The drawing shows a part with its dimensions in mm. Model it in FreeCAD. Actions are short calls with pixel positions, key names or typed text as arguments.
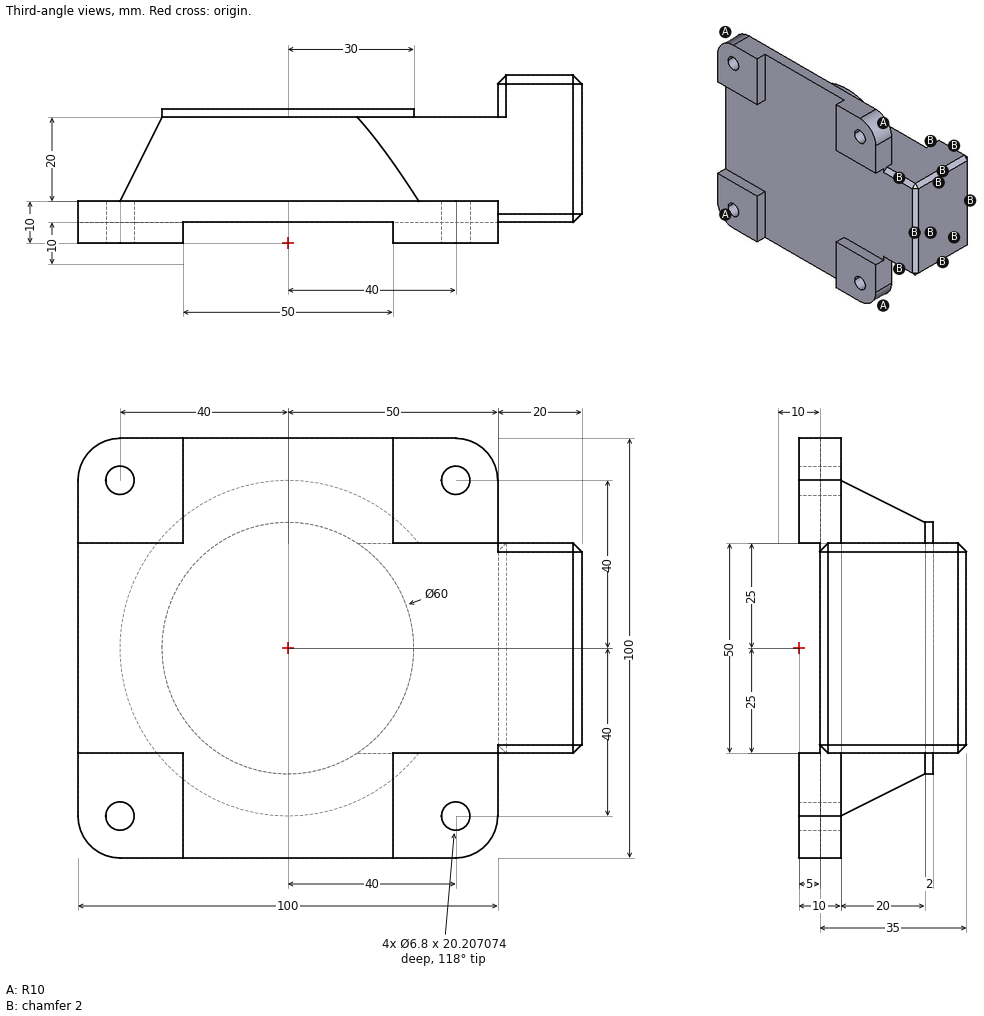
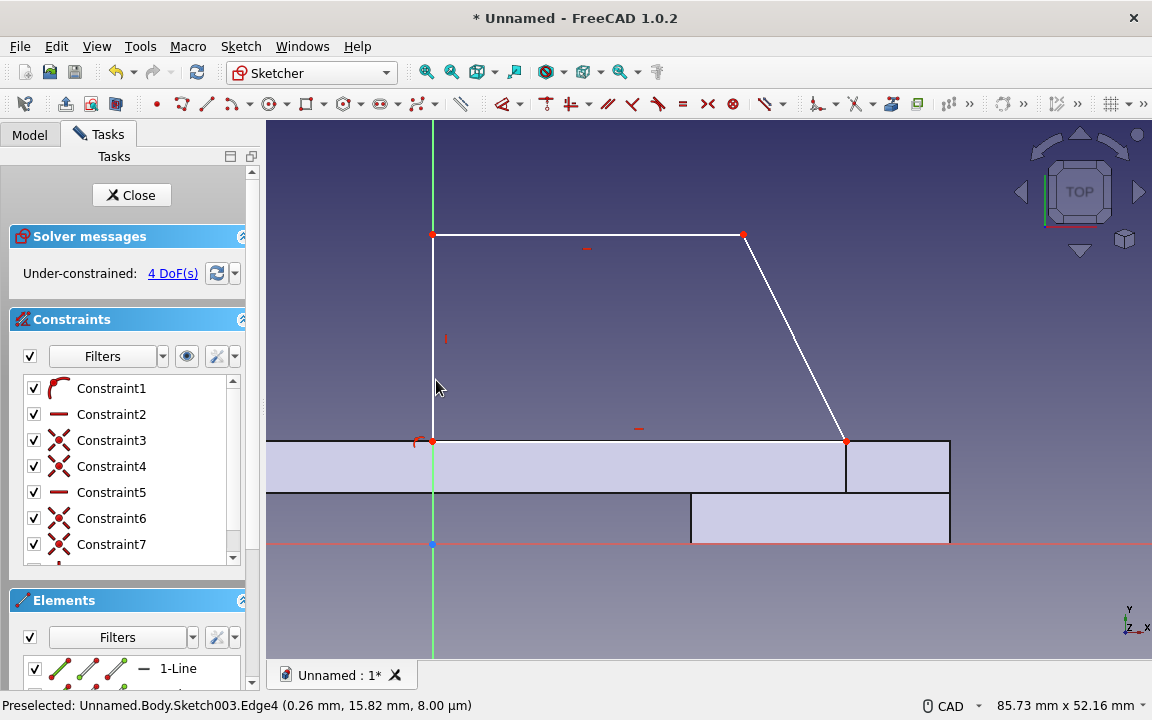
key(d)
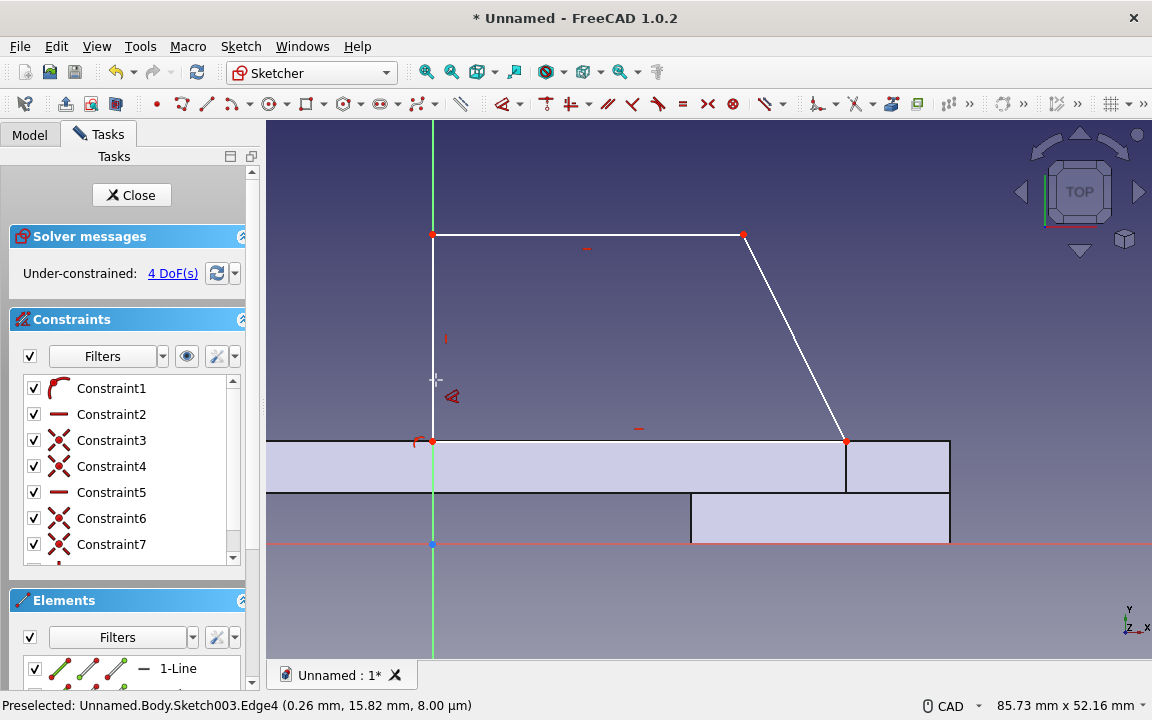
click(557, 442)
click(639, 476)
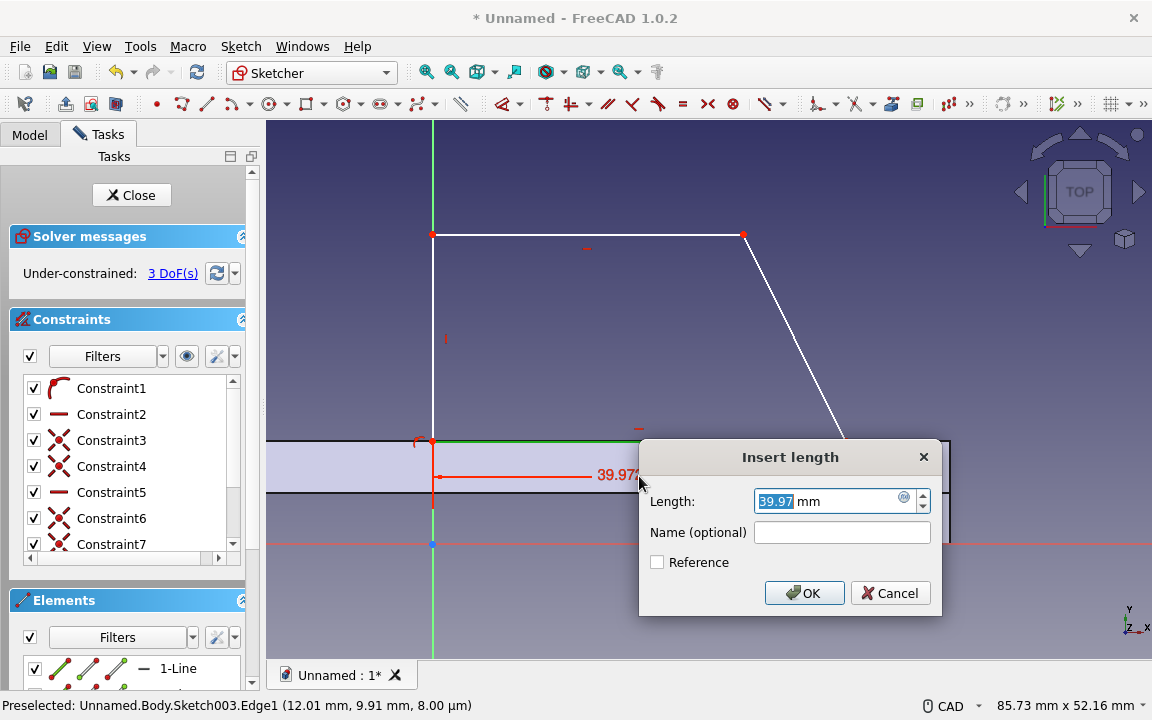
text(40)
key(Return)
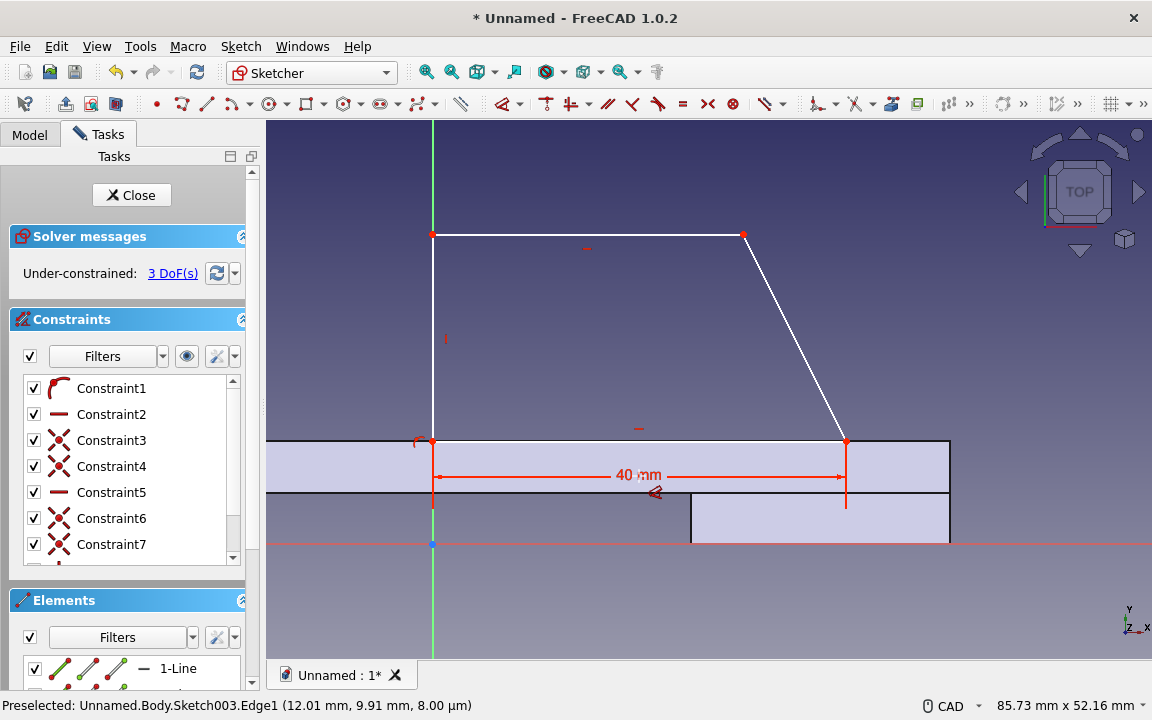
click(650, 235)
click(588, 201)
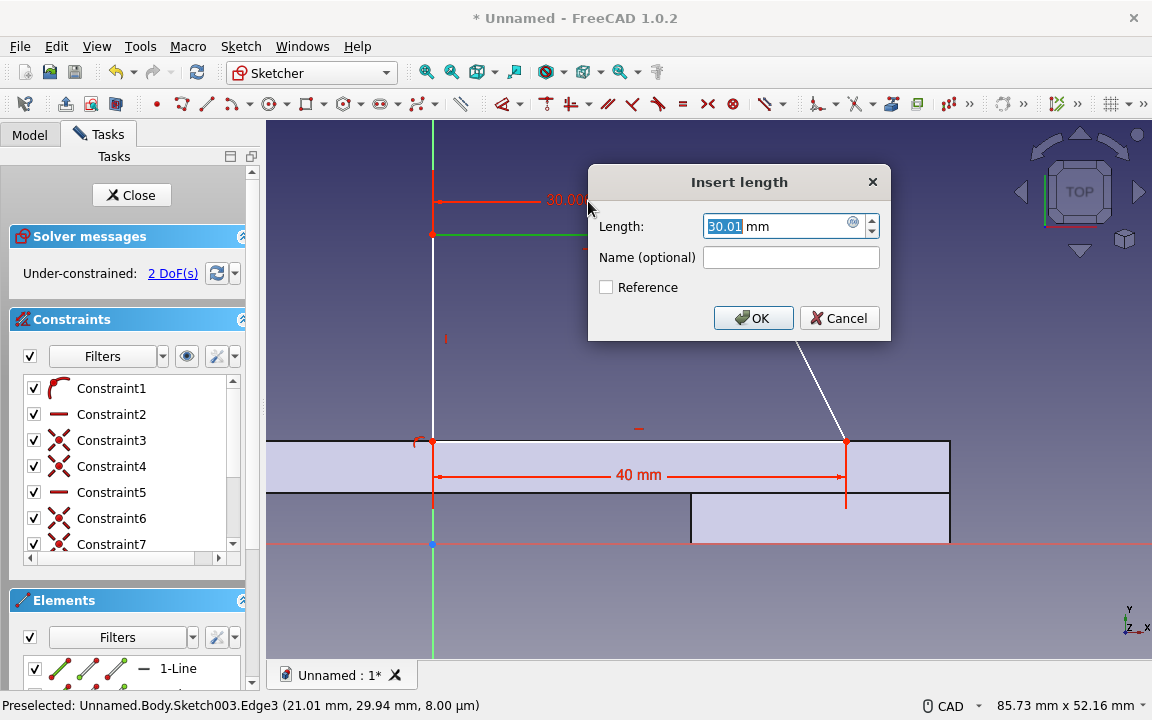
text(30)
key(Return)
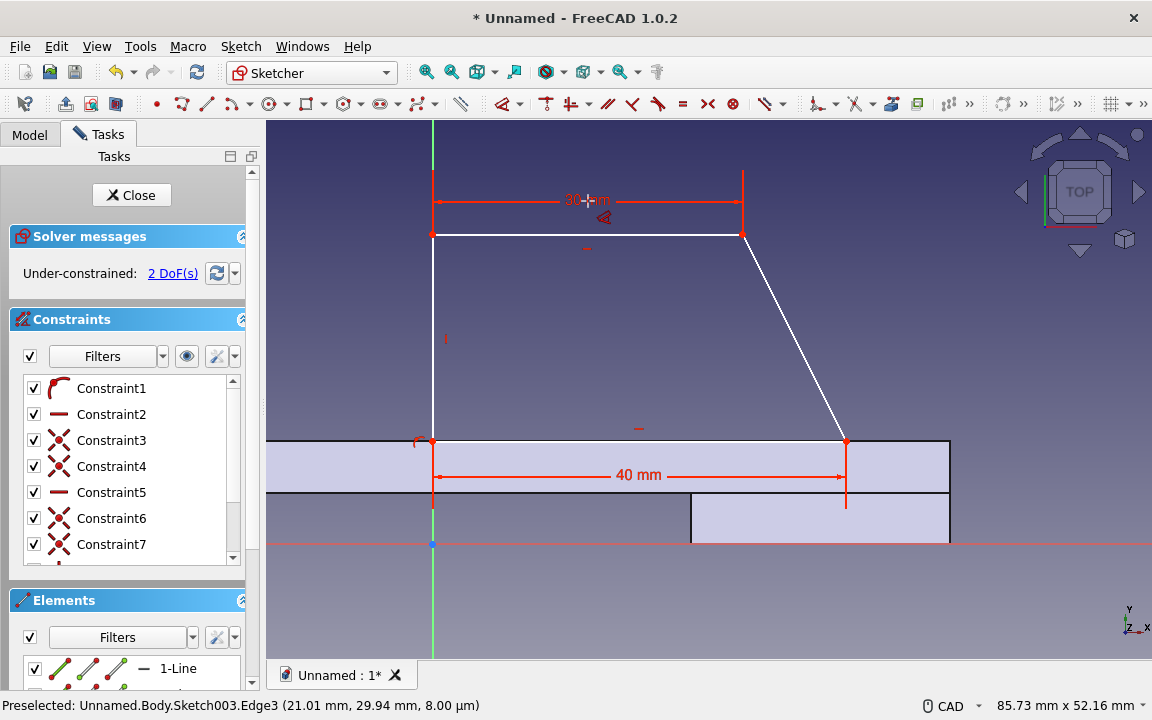
click(433, 297)
click(399, 338)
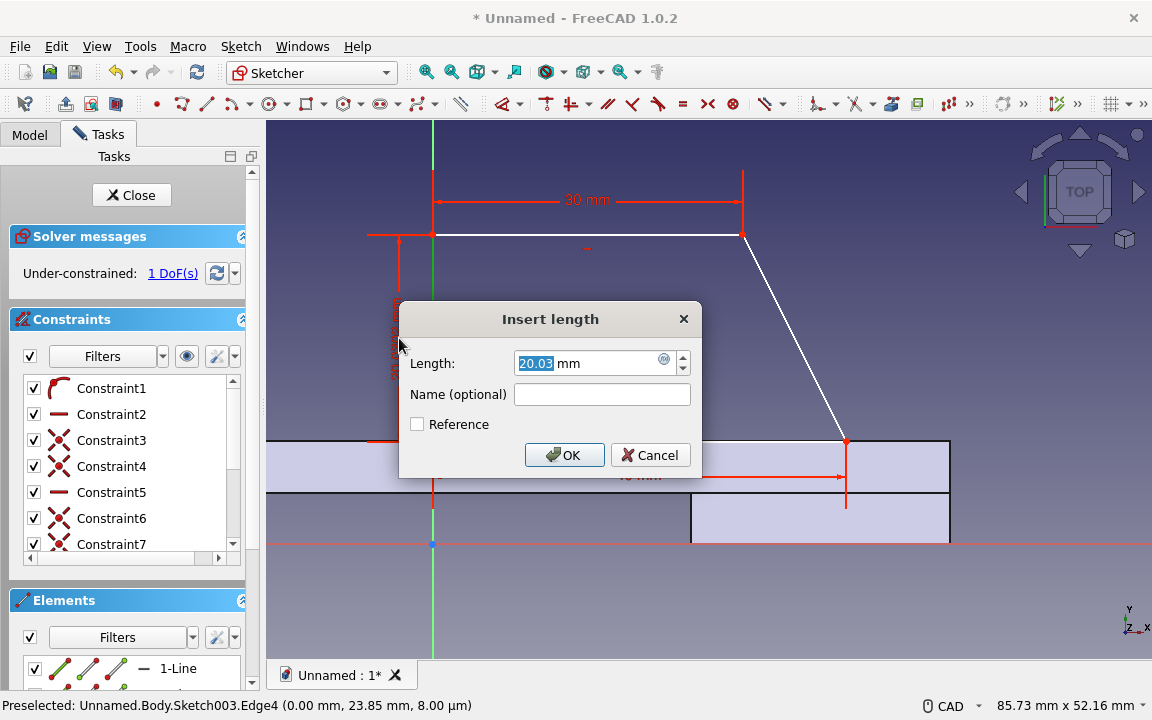
text(20)
key(Return)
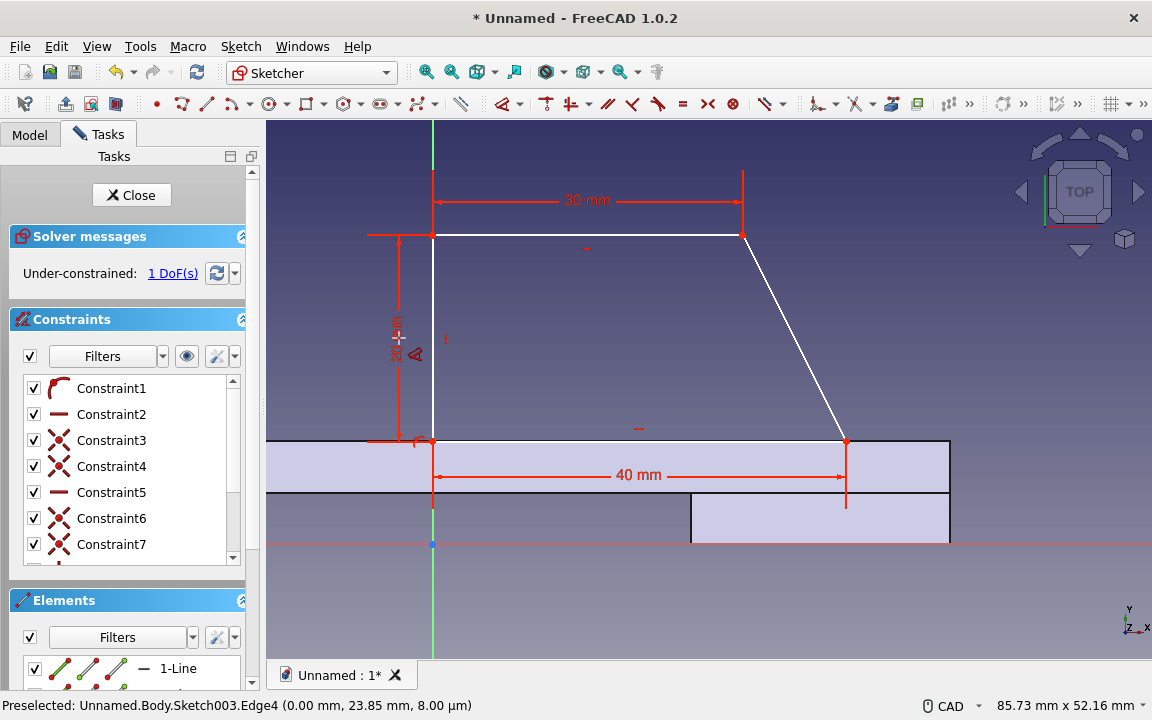
click(433, 442)
click(399, 493)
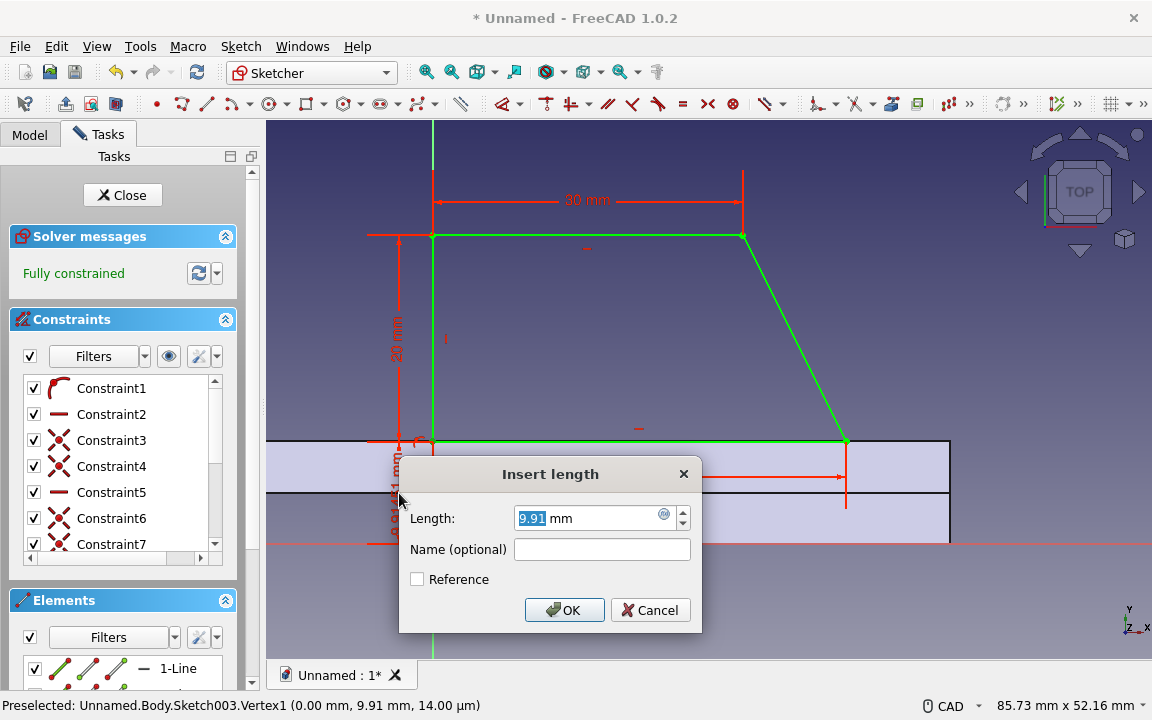
text(10)
key(Return)
key(Escape)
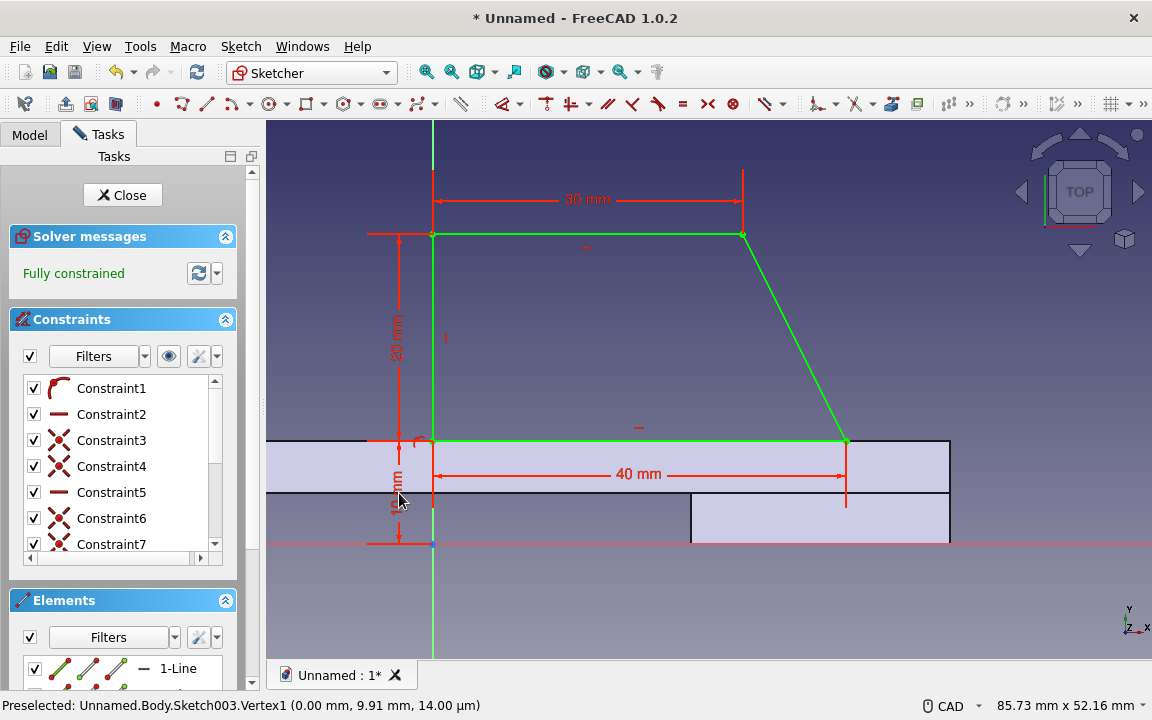
click(123, 195)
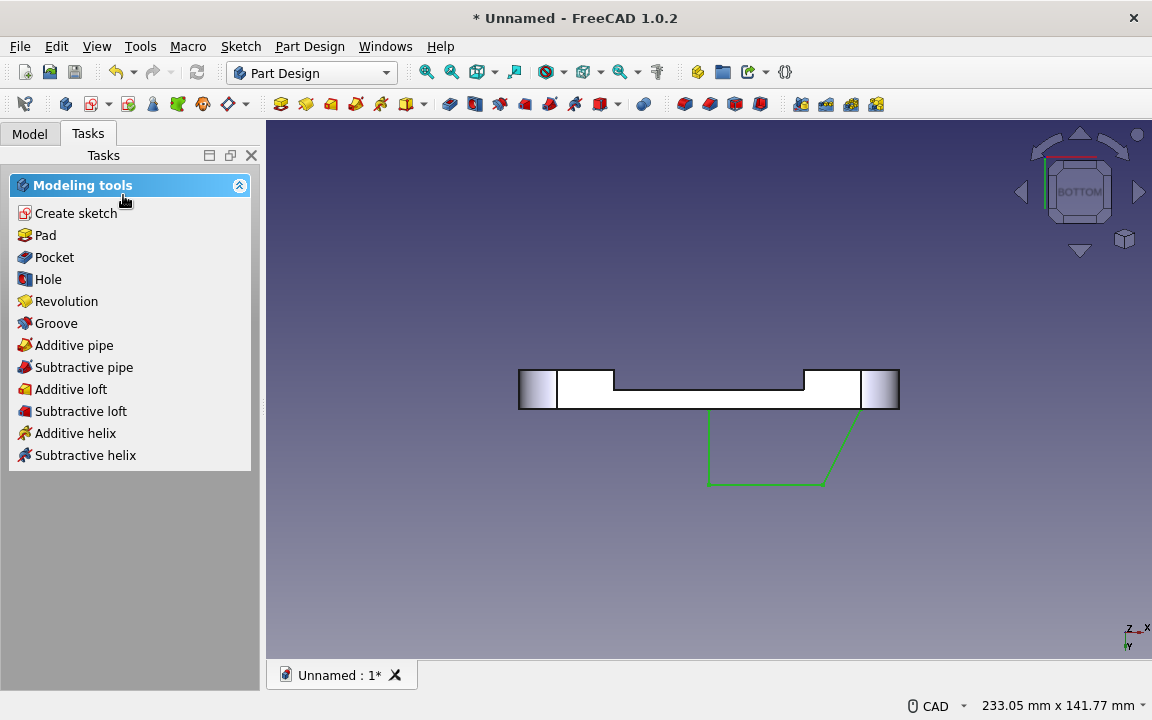
click(306, 104)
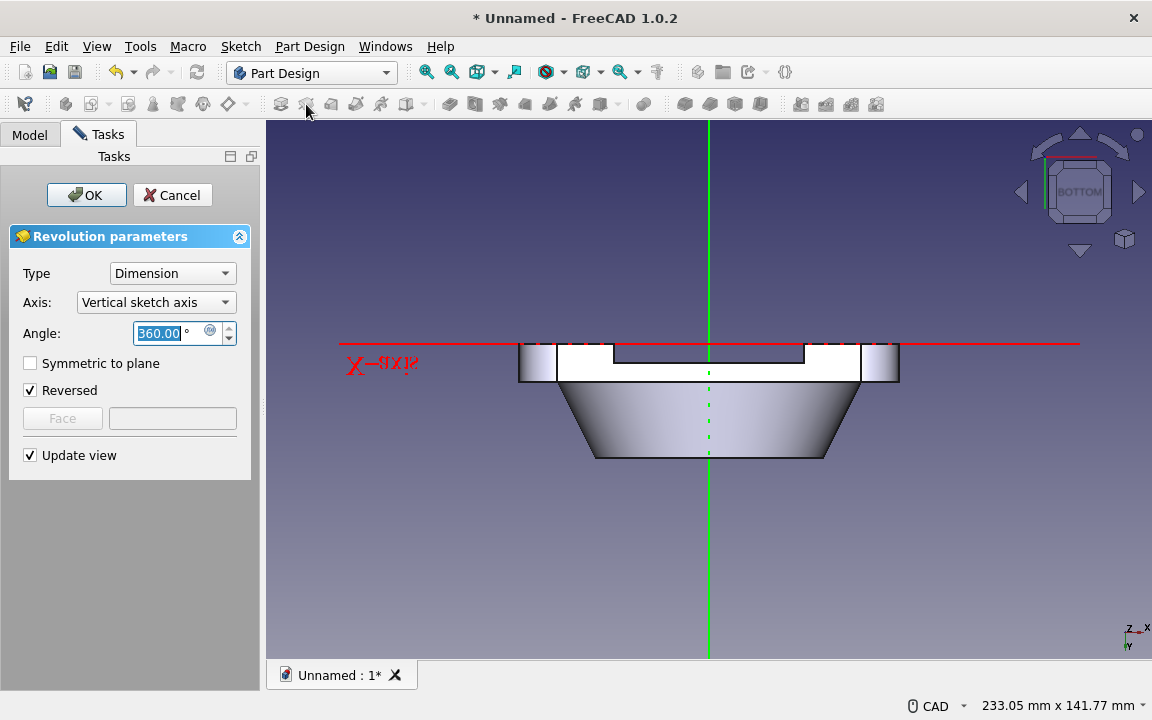
click(87, 195)